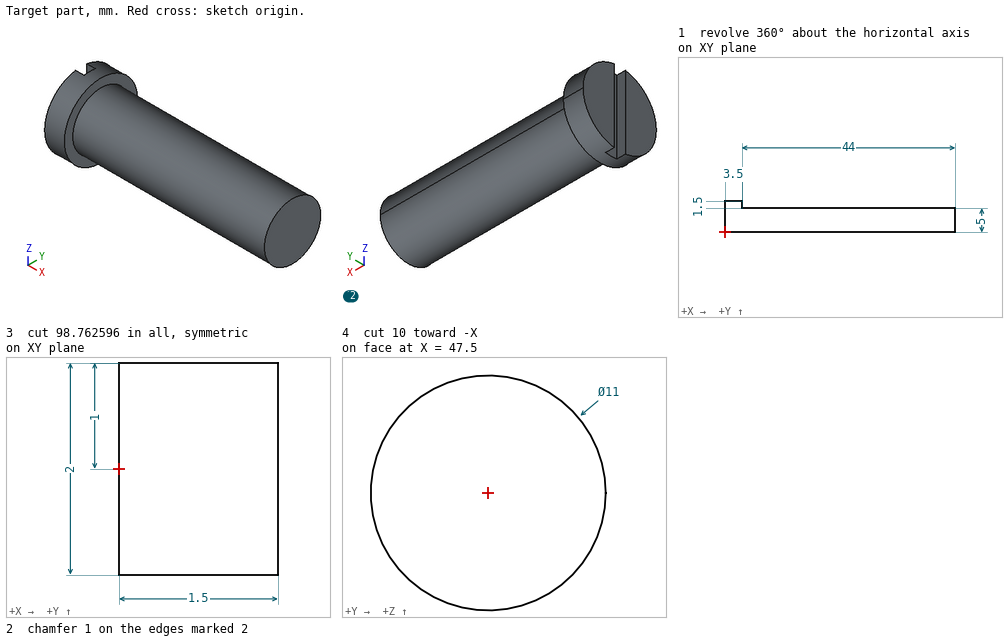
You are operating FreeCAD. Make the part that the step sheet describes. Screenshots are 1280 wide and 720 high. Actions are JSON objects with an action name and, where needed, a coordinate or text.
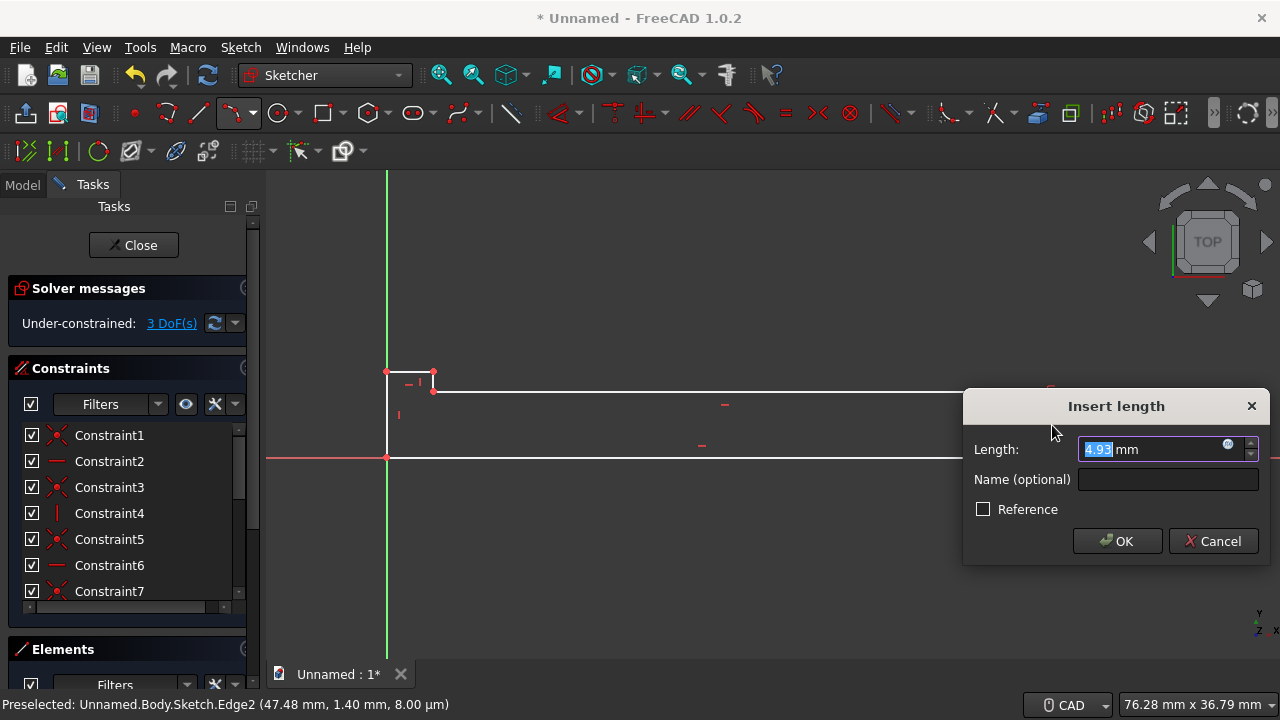
{"action": "type", "text": "5"}
{"action": "key", "text": "Return"}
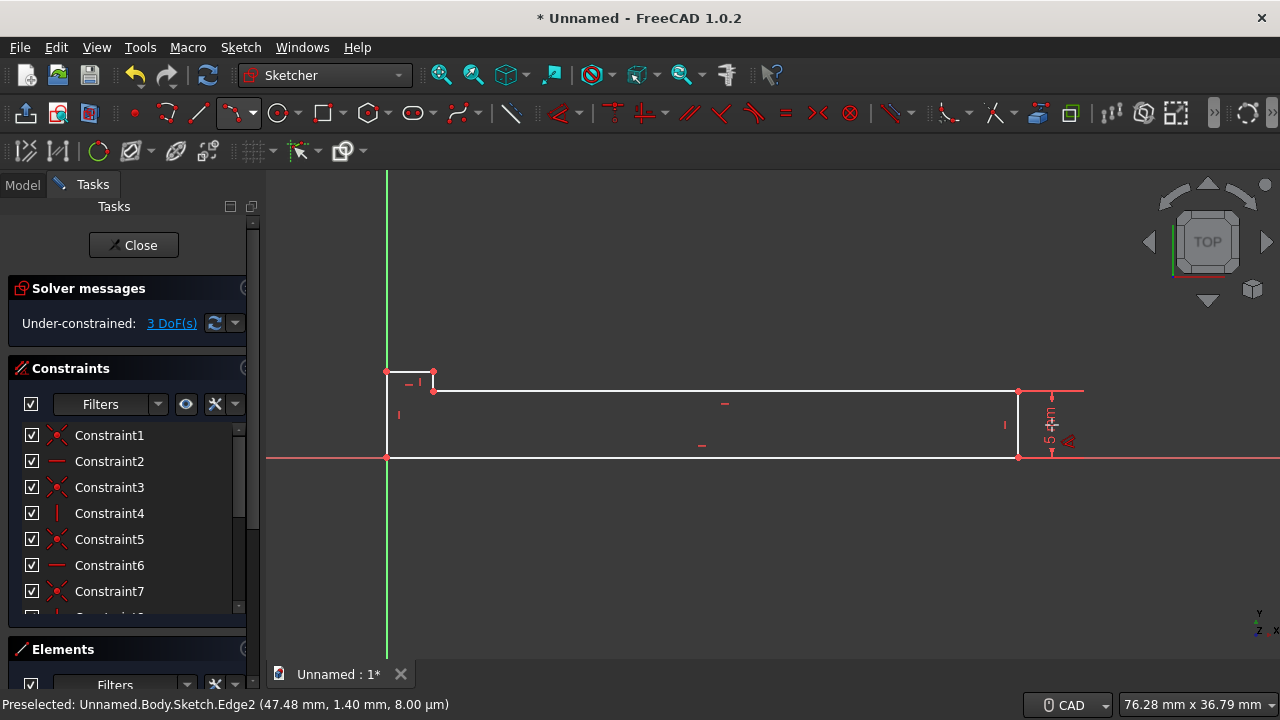
{"action": "left_click", "coordinate": [843, 391]}
{"action": "left_click", "coordinate": [726, 357]}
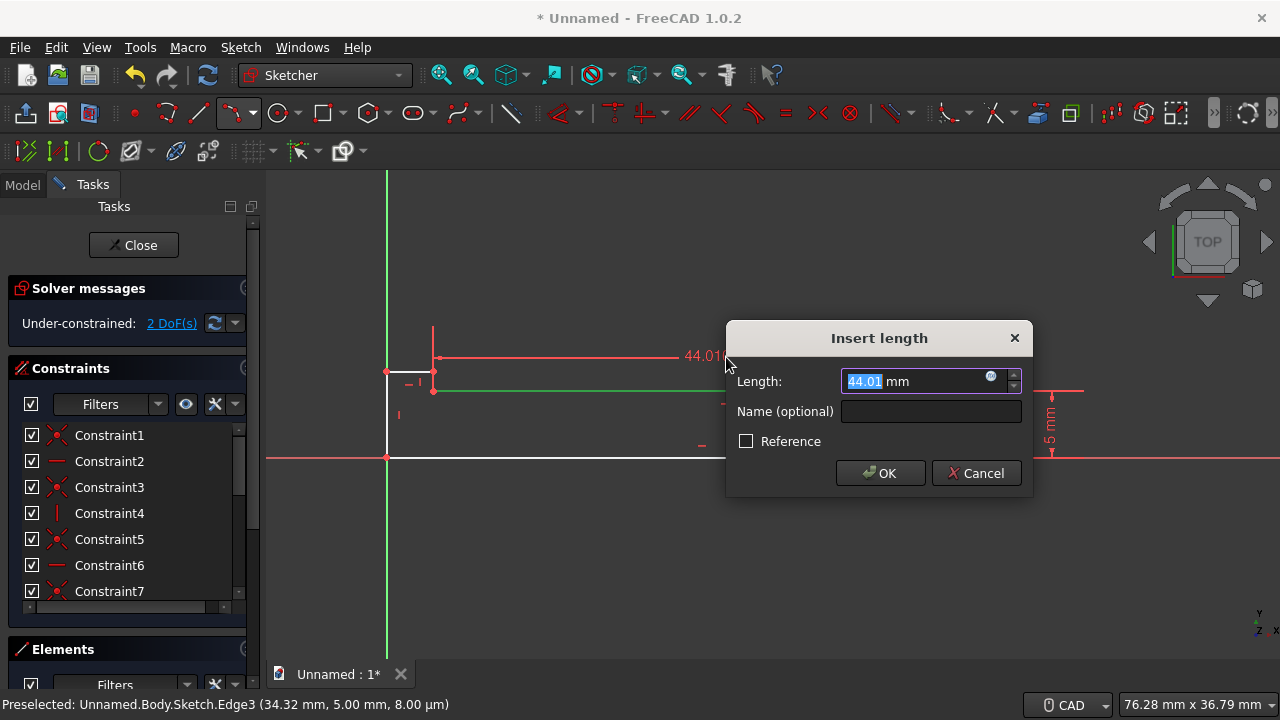
{"action": "type", "text": "44"}
{"action": "key", "text": "Return"}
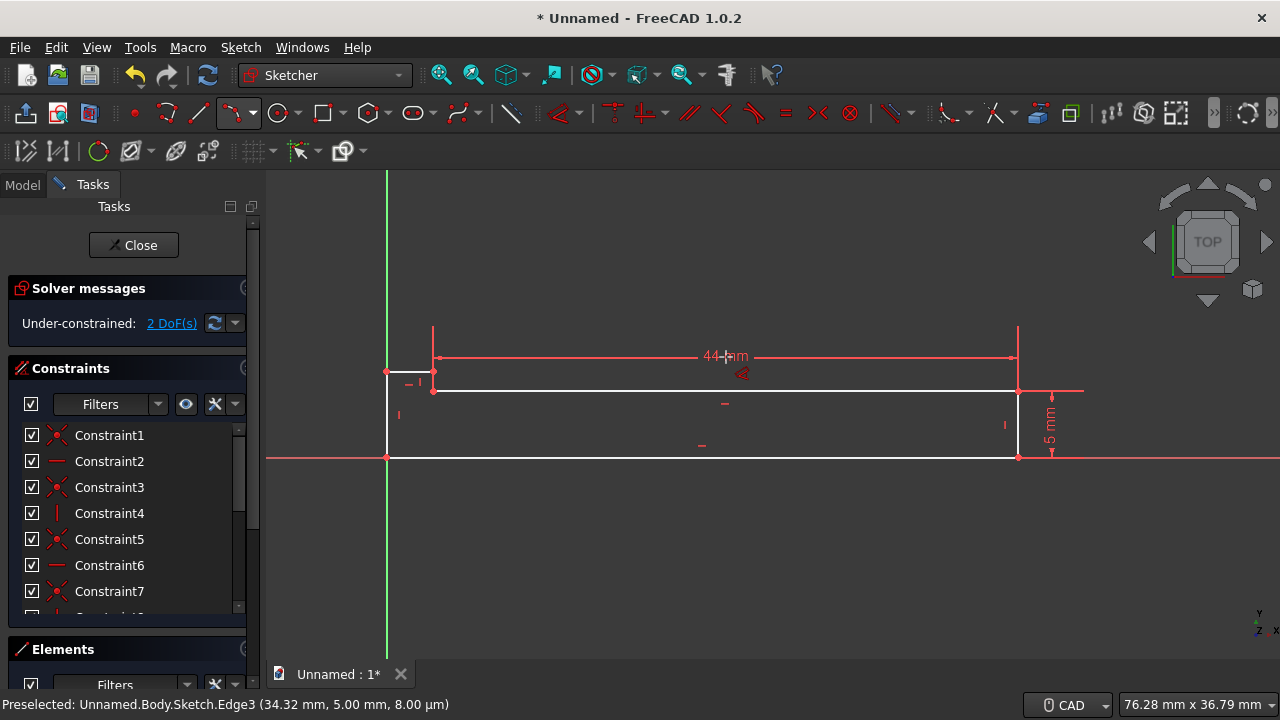
{"action": "scroll", "coordinate": [433, 382], "scroll_direction": "up", "scroll_amount": 4}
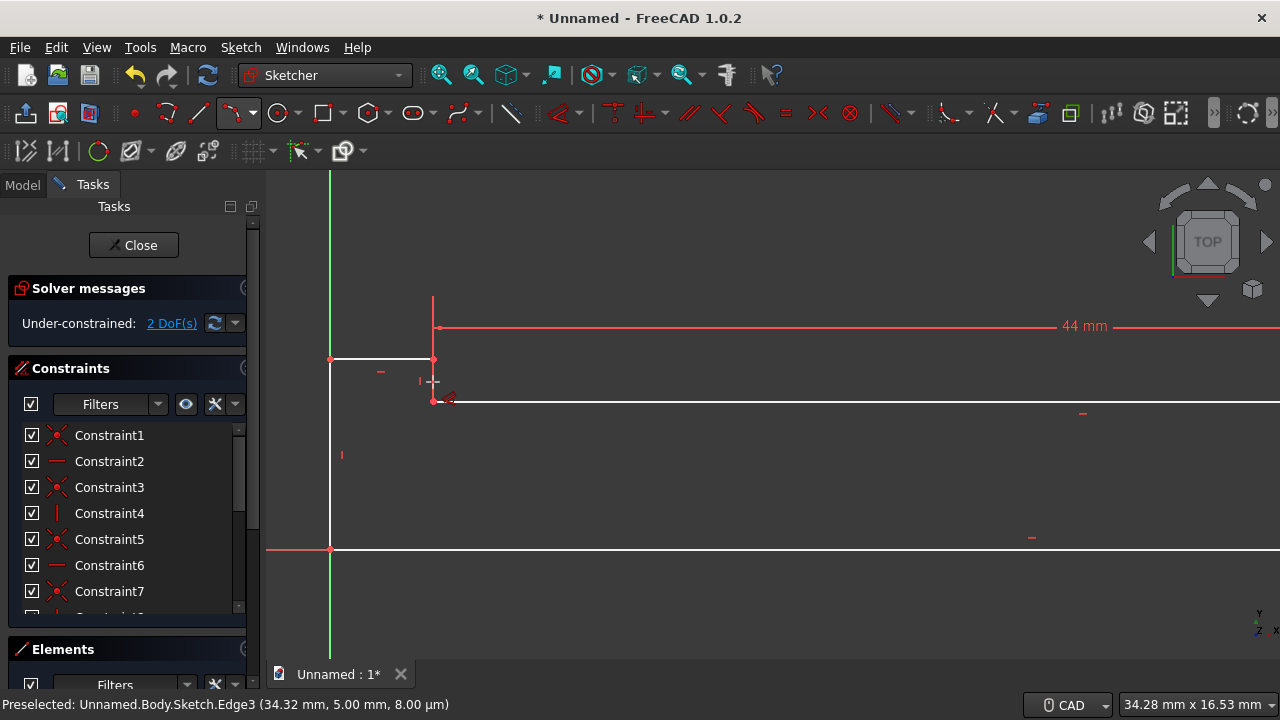
{"action": "left_click", "coordinate": [433, 380]}
{"action": "left_click", "coordinate": [399, 380]}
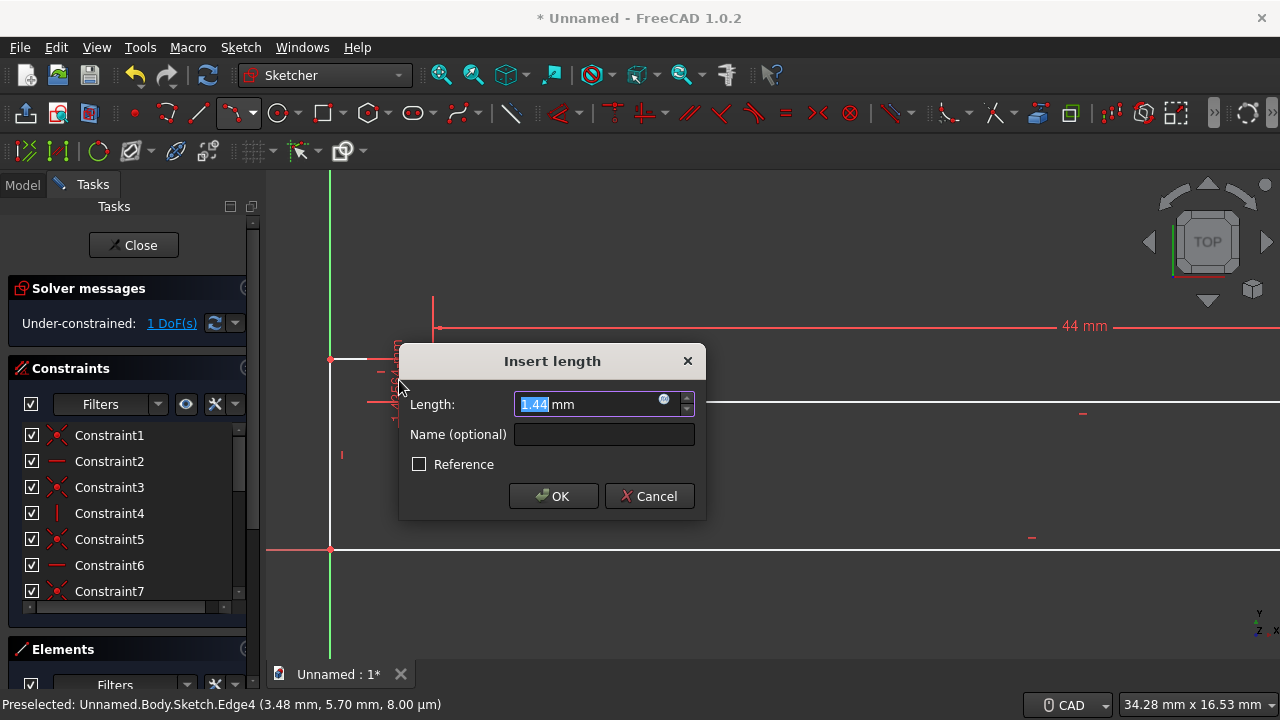
{"action": "type", "text": "1.5"}
{"action": "key", "text": "Return"}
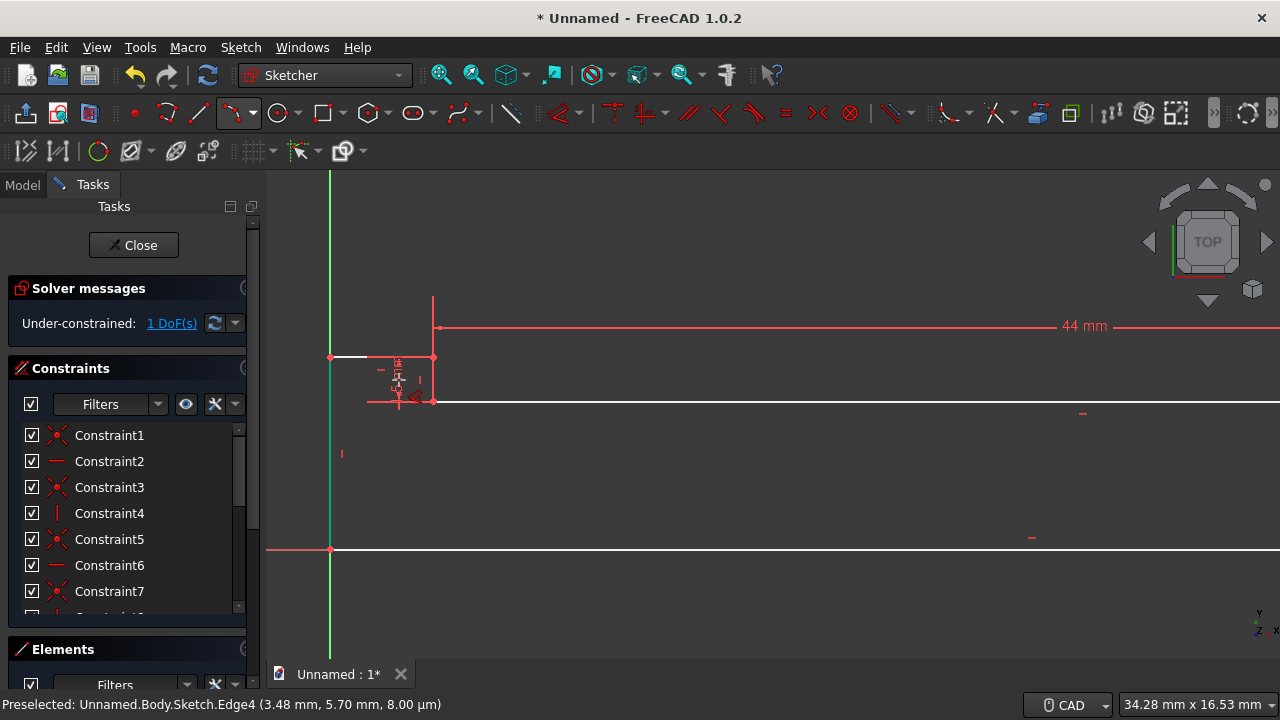
{"action": "left_click", "coordinate": [402, 357]}
{"action": "left_click", "coordinate": [382, 323]}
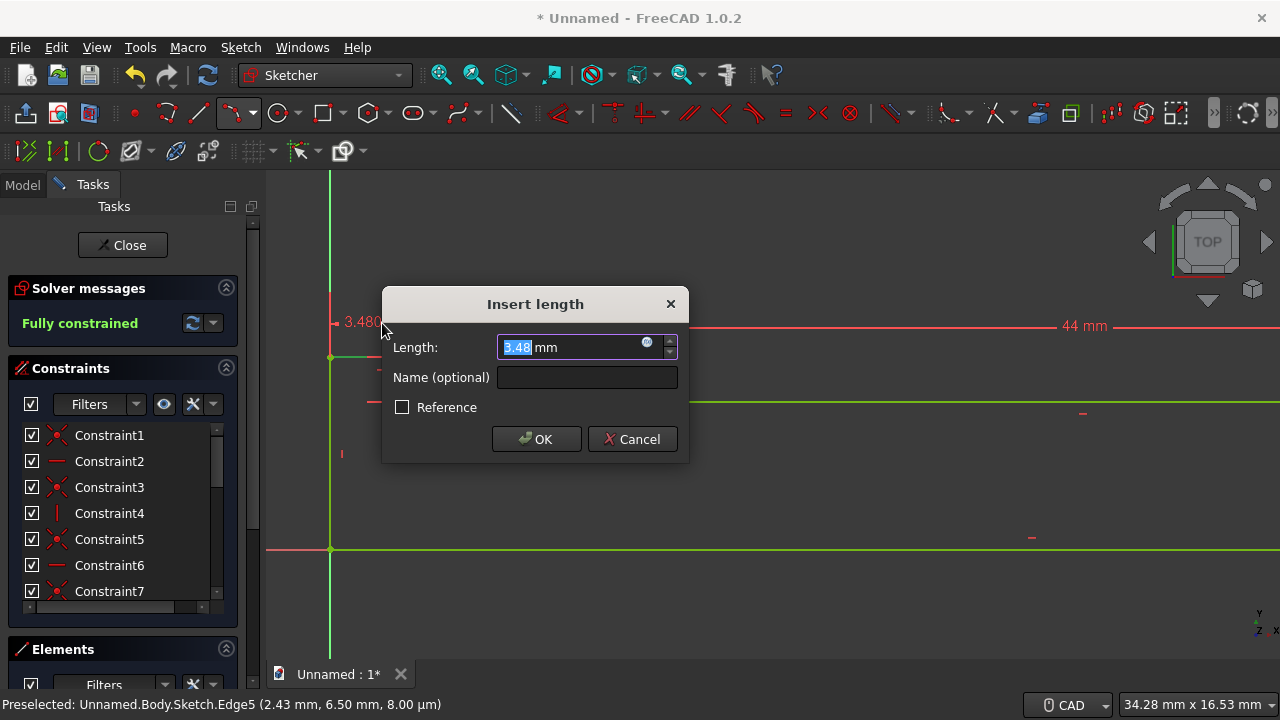
{"action": "type", "text": "3.5"}
{"action": "key", "text": "Return"}
{"action": "key", "text": "Escape"}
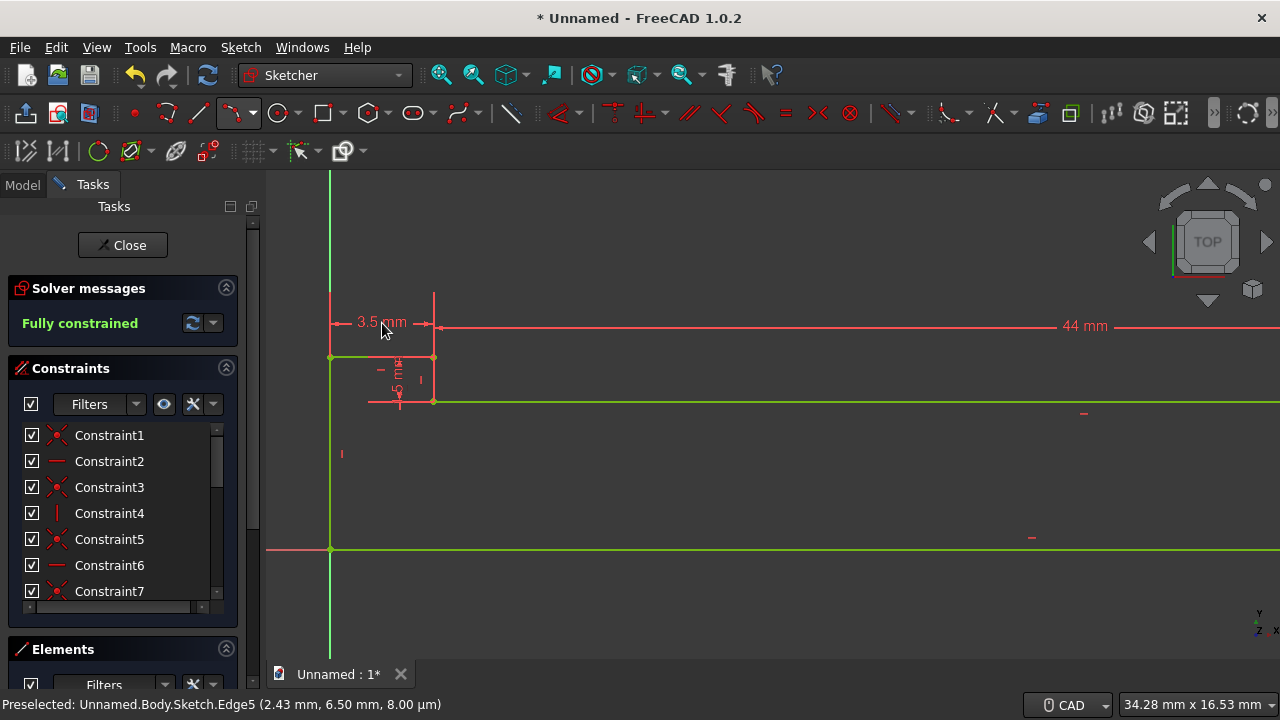
{"action": "left_click", "coordinate": [123, 245]}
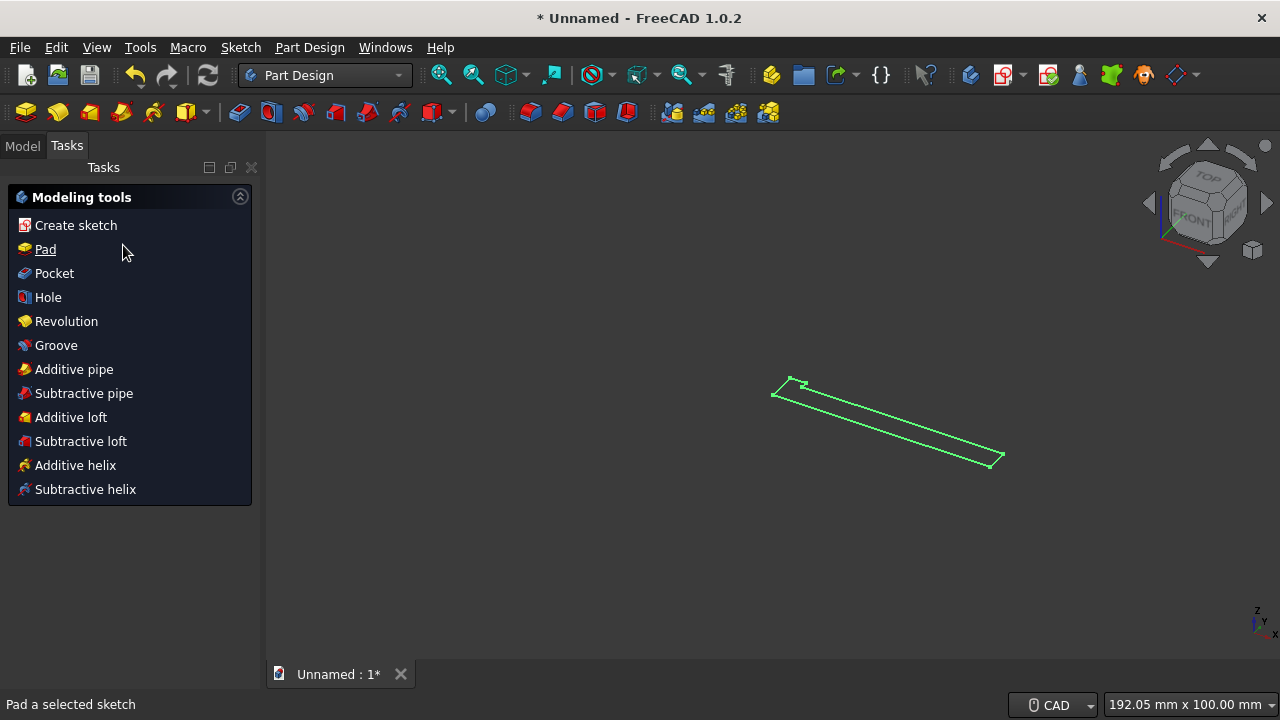
{"action": "left_click", "coordinate": [58, 112]}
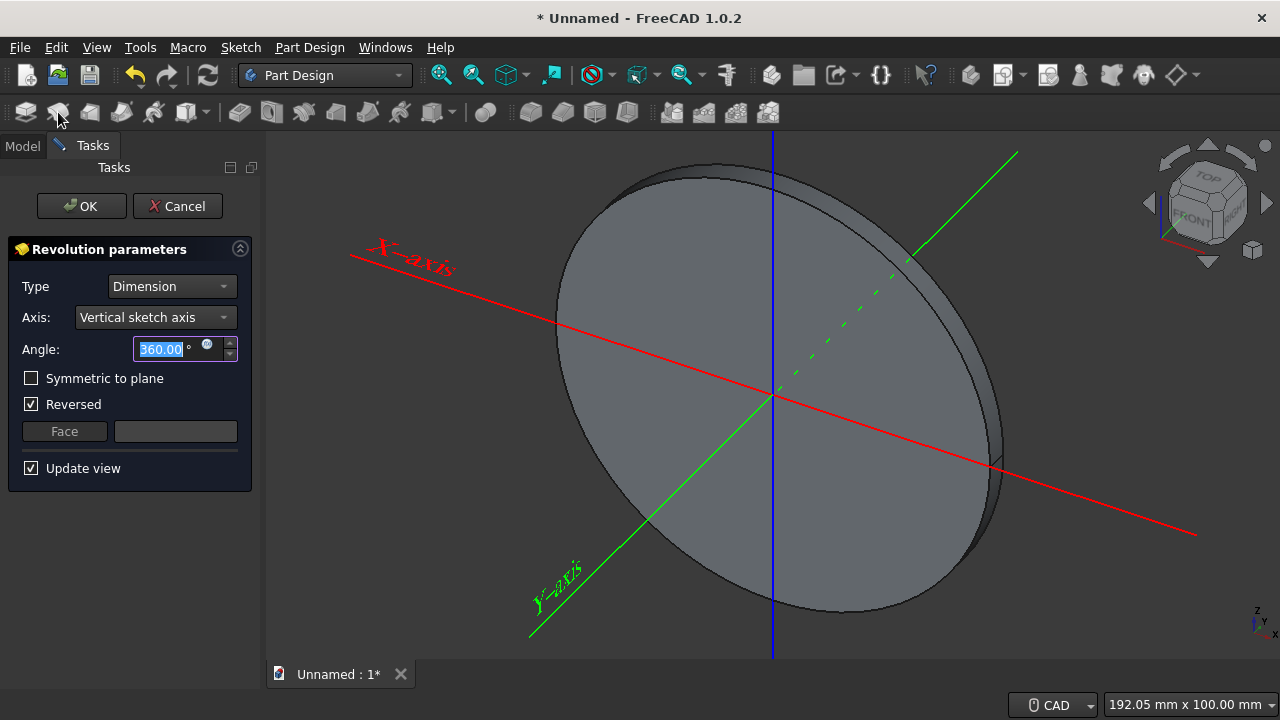
{"action": "left_click", "coordinate": [156, 318]}